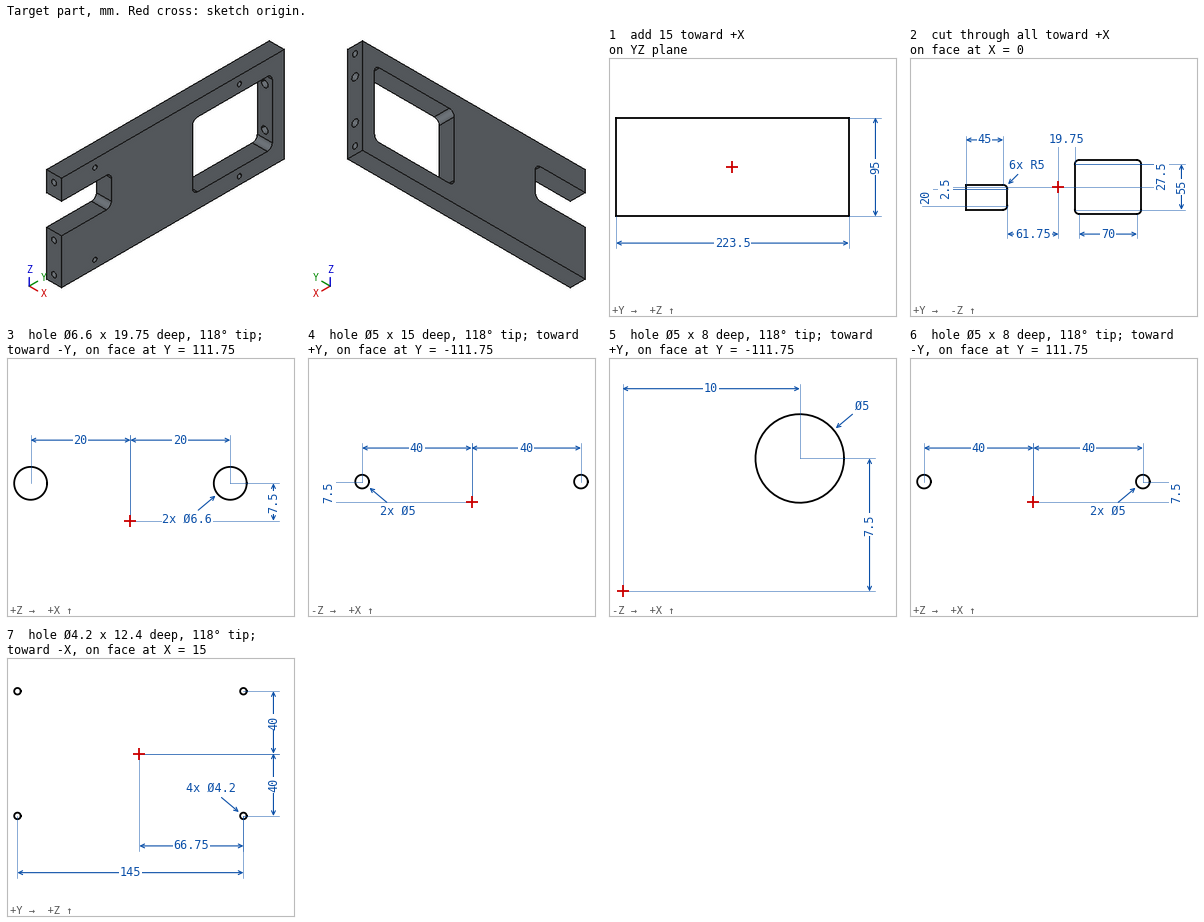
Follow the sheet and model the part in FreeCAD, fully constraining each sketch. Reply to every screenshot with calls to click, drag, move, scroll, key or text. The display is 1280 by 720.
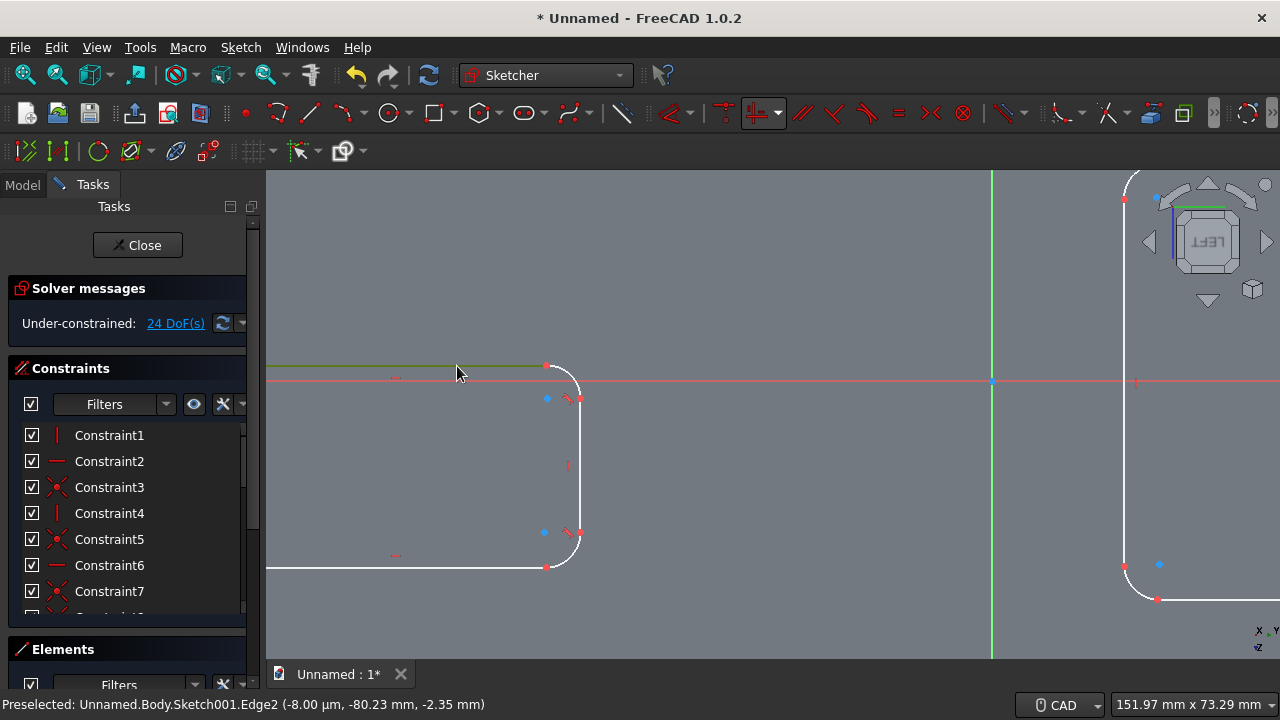
click(577, 383)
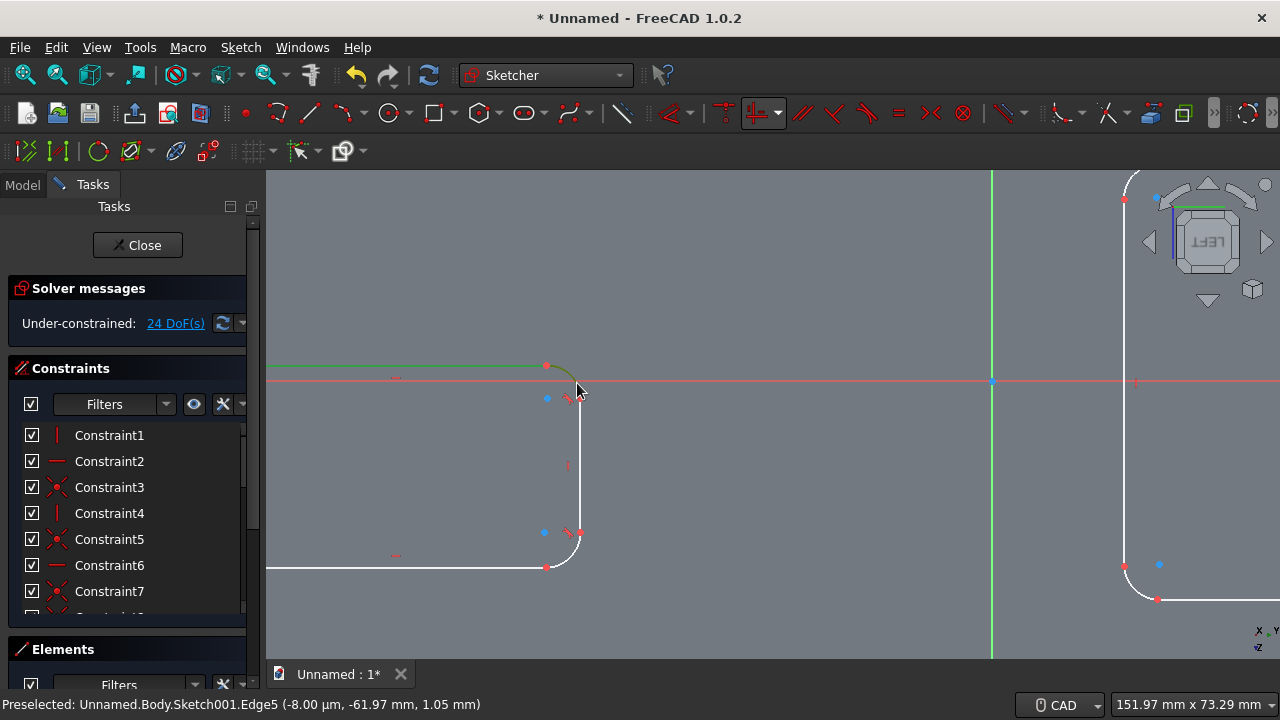
click(868, 114)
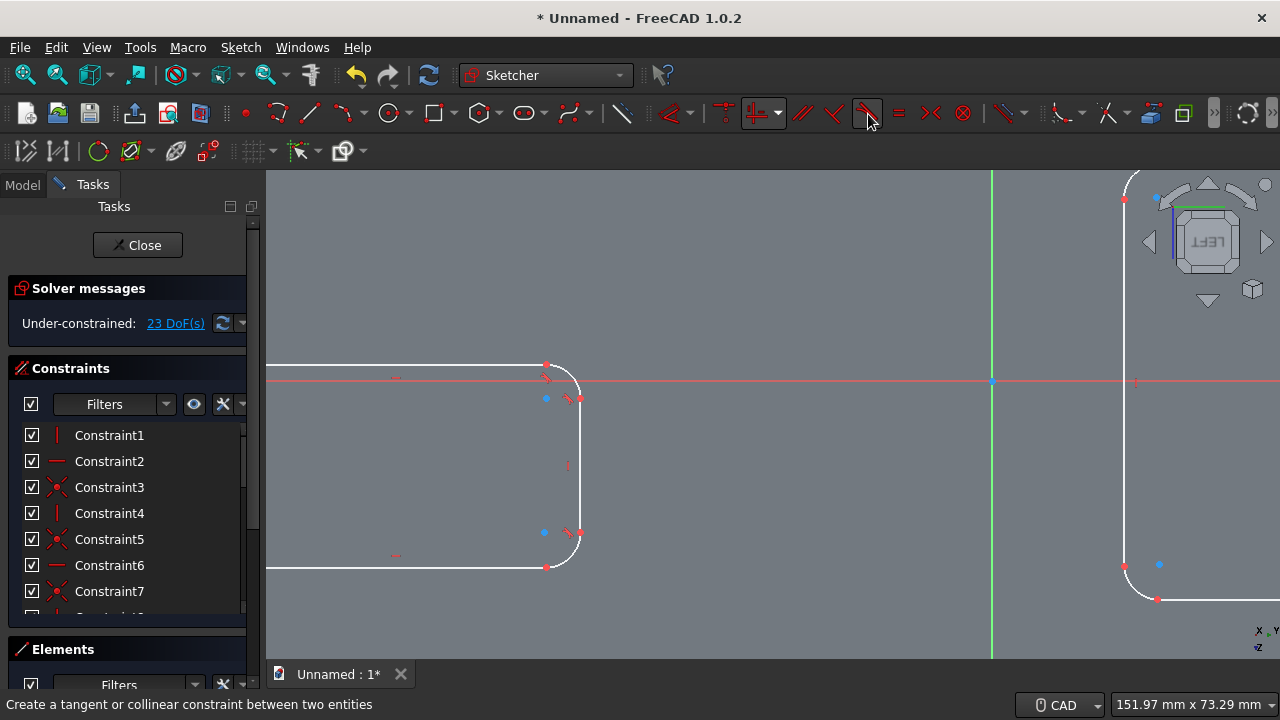
click(337, 568)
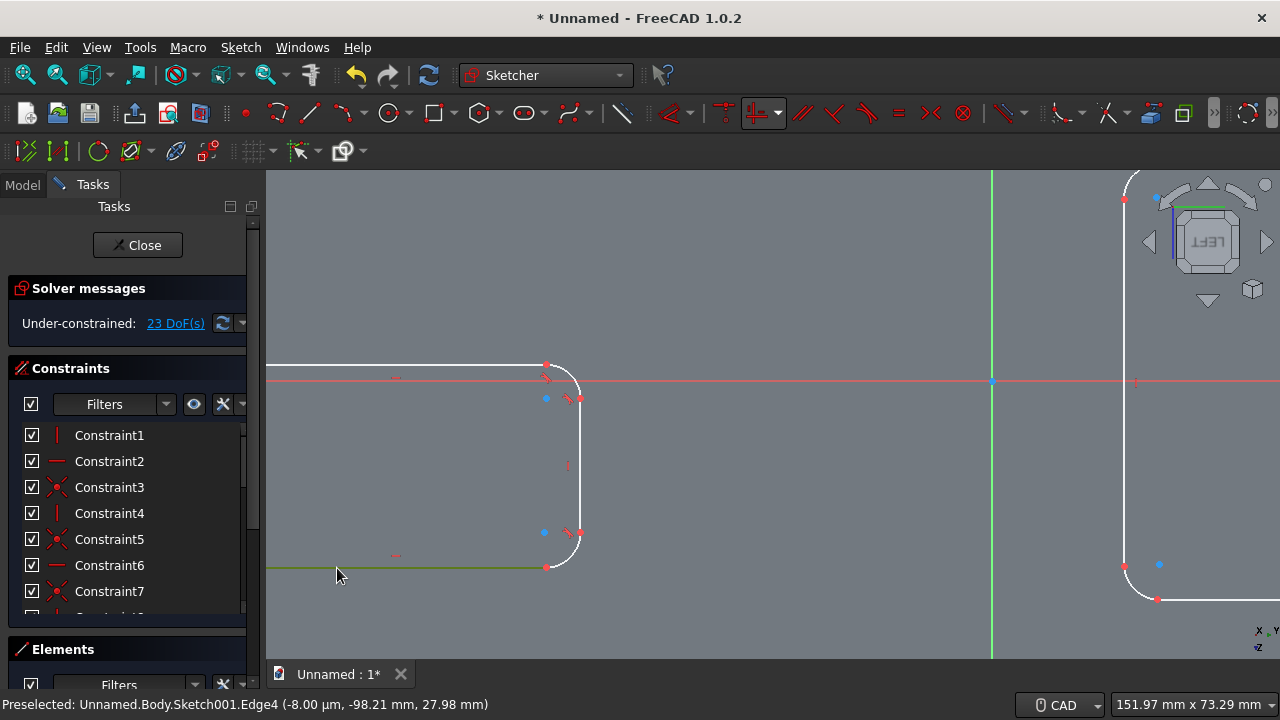
click(562, 563)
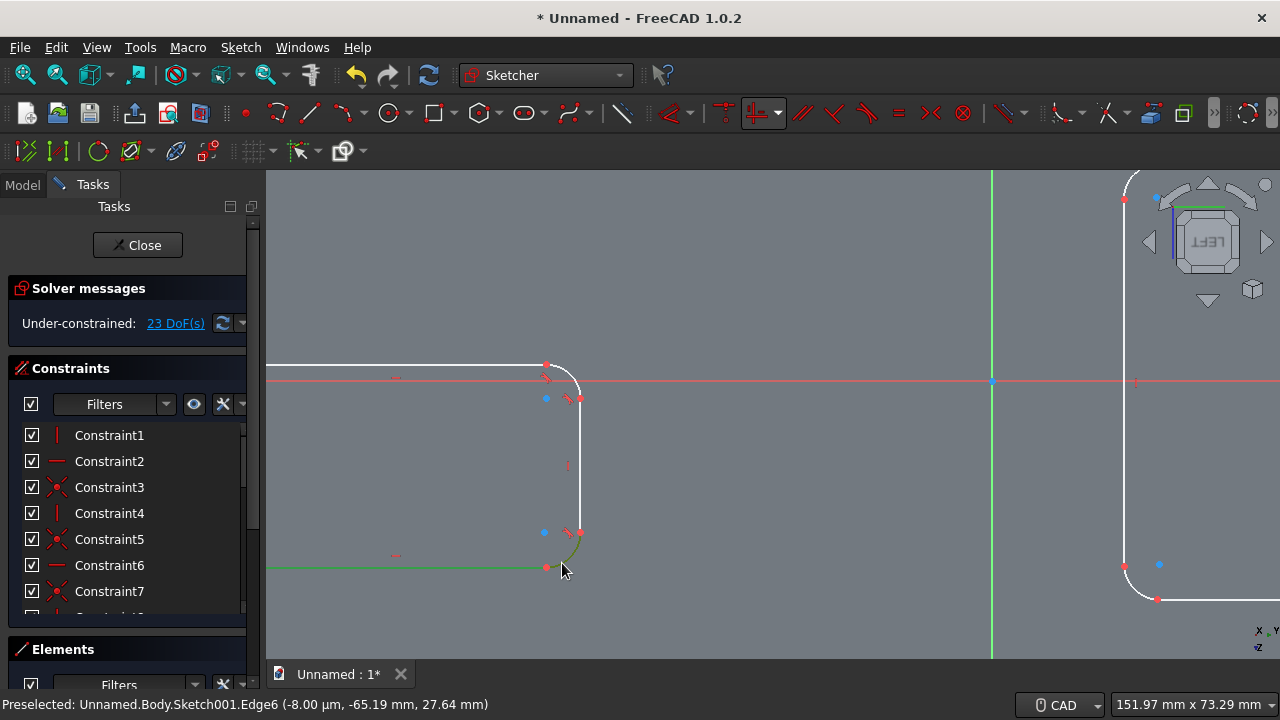
click(868, 114)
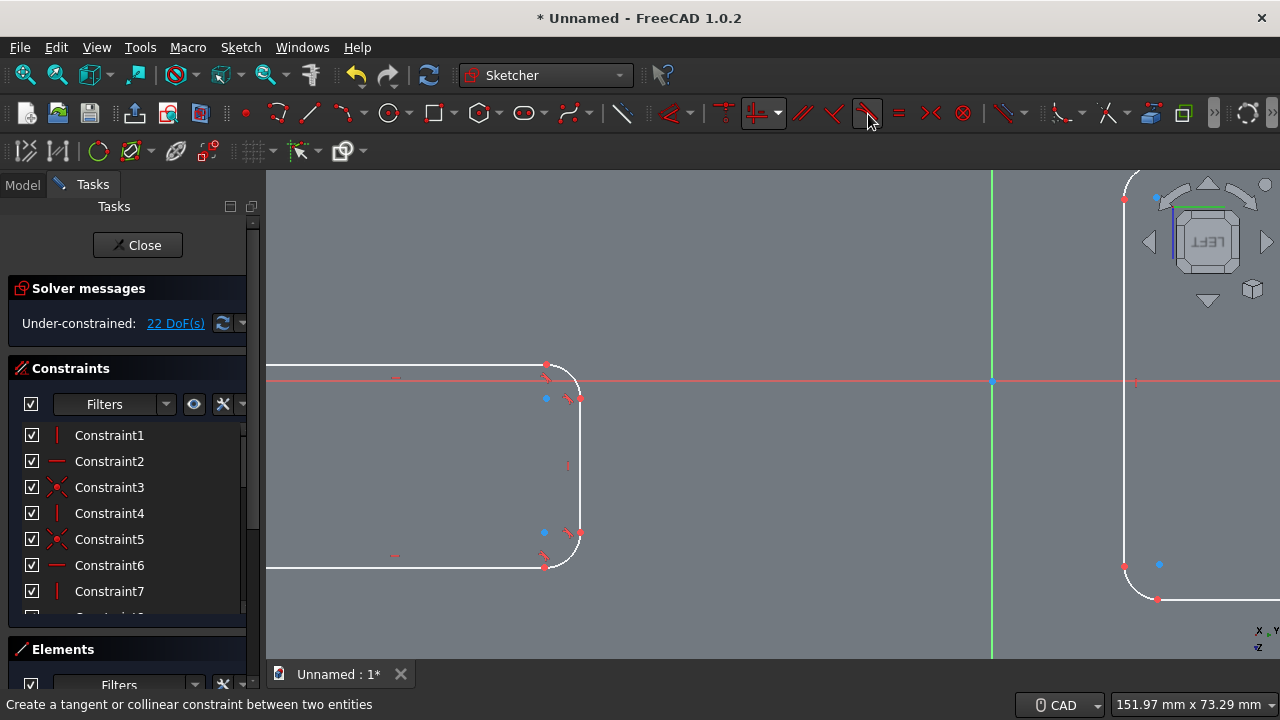
scroll(502, 442, down, 4)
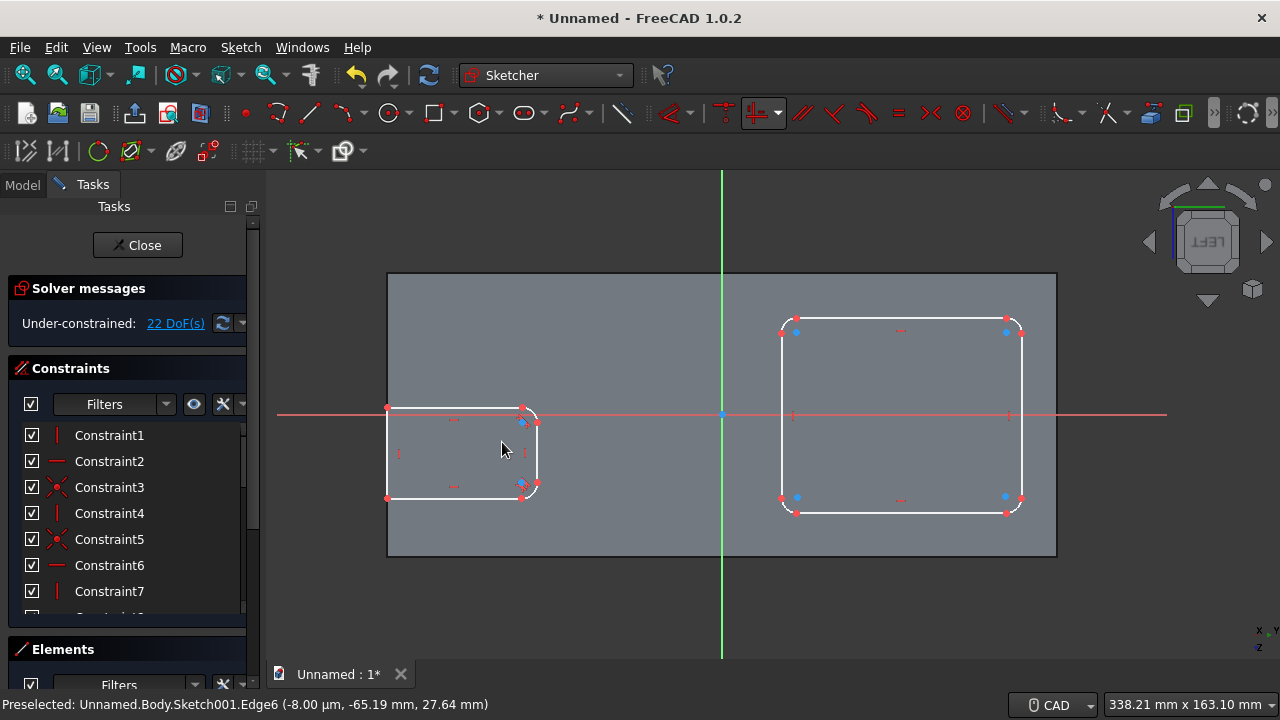
click(782, 383)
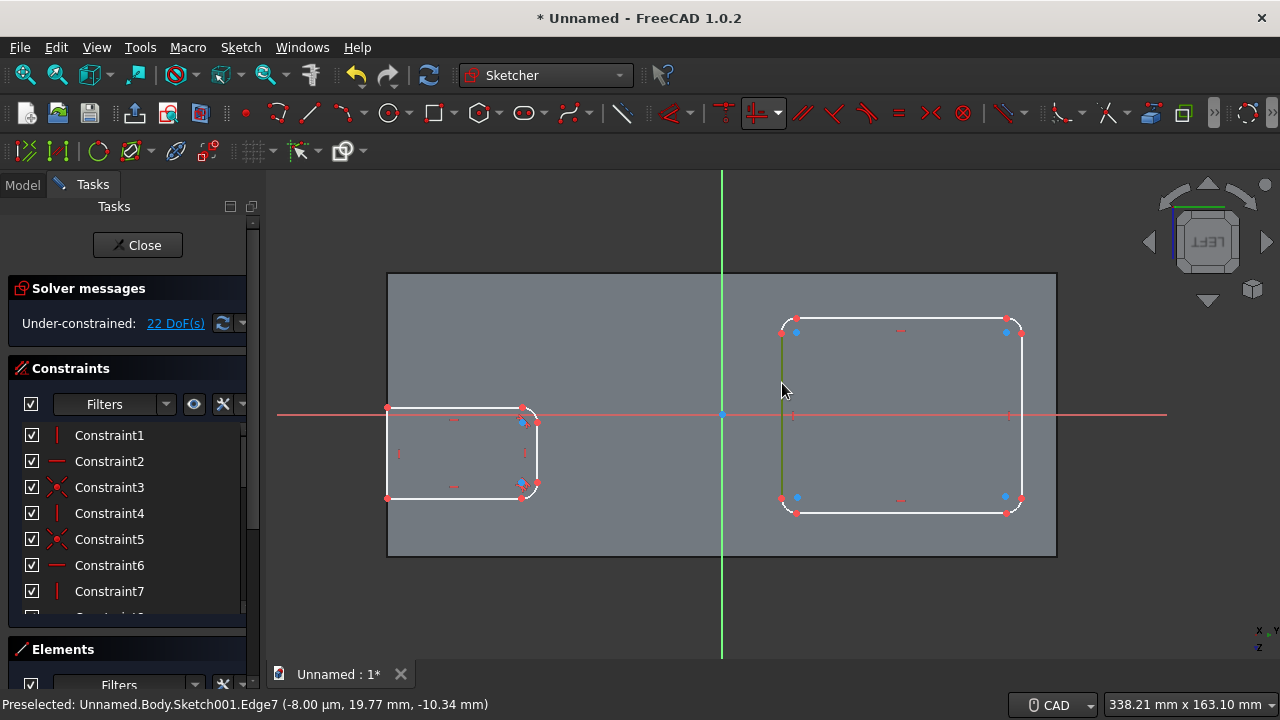
click(786, 509)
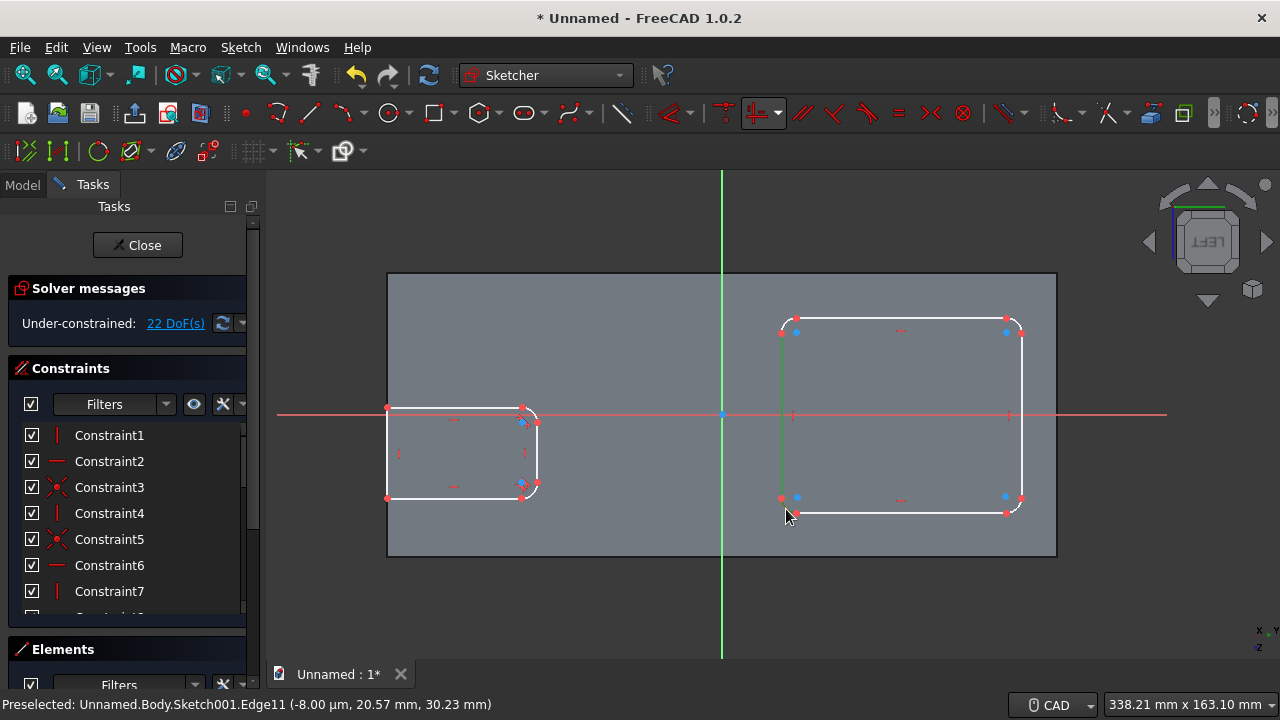
click(868, 114)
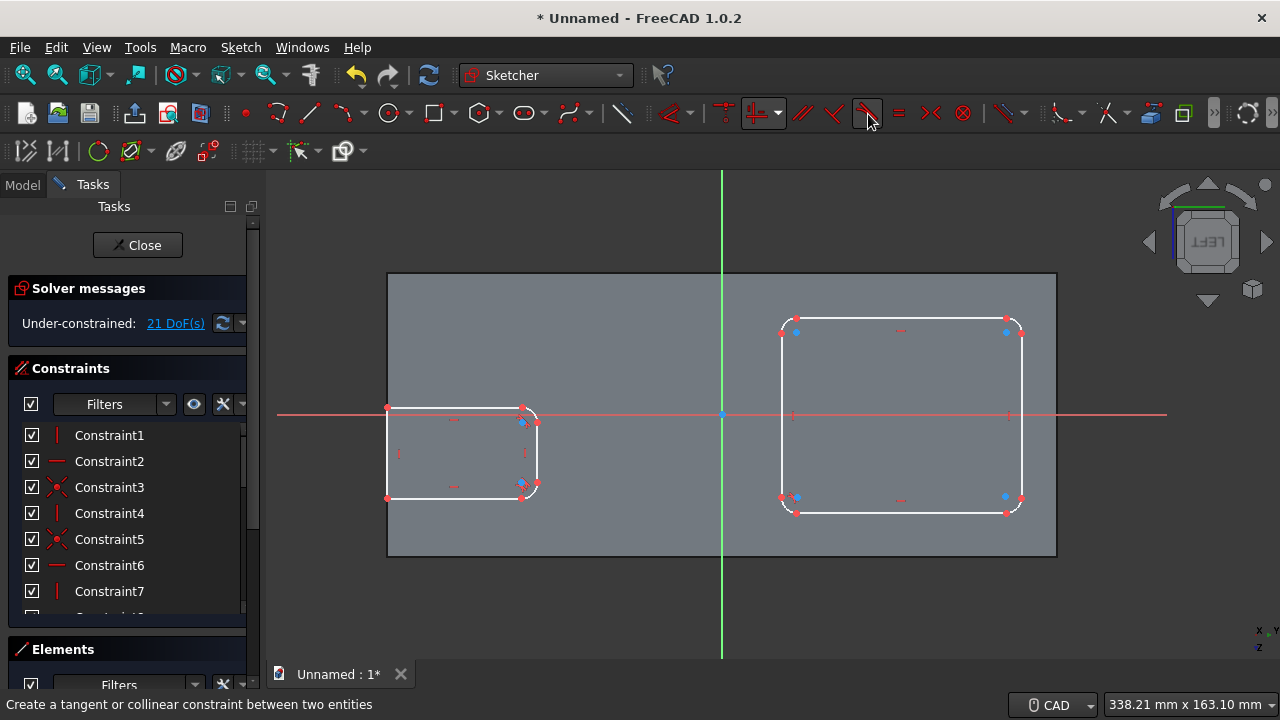
click(782, 382)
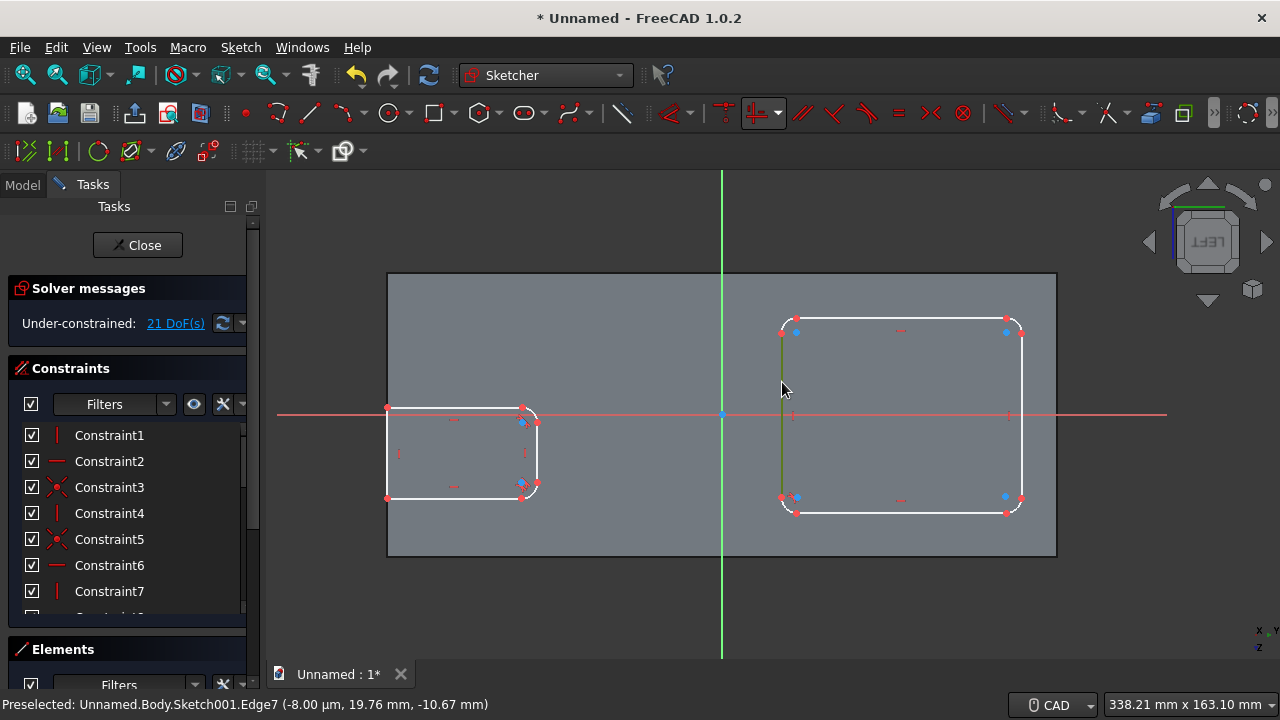
click(786, 322)